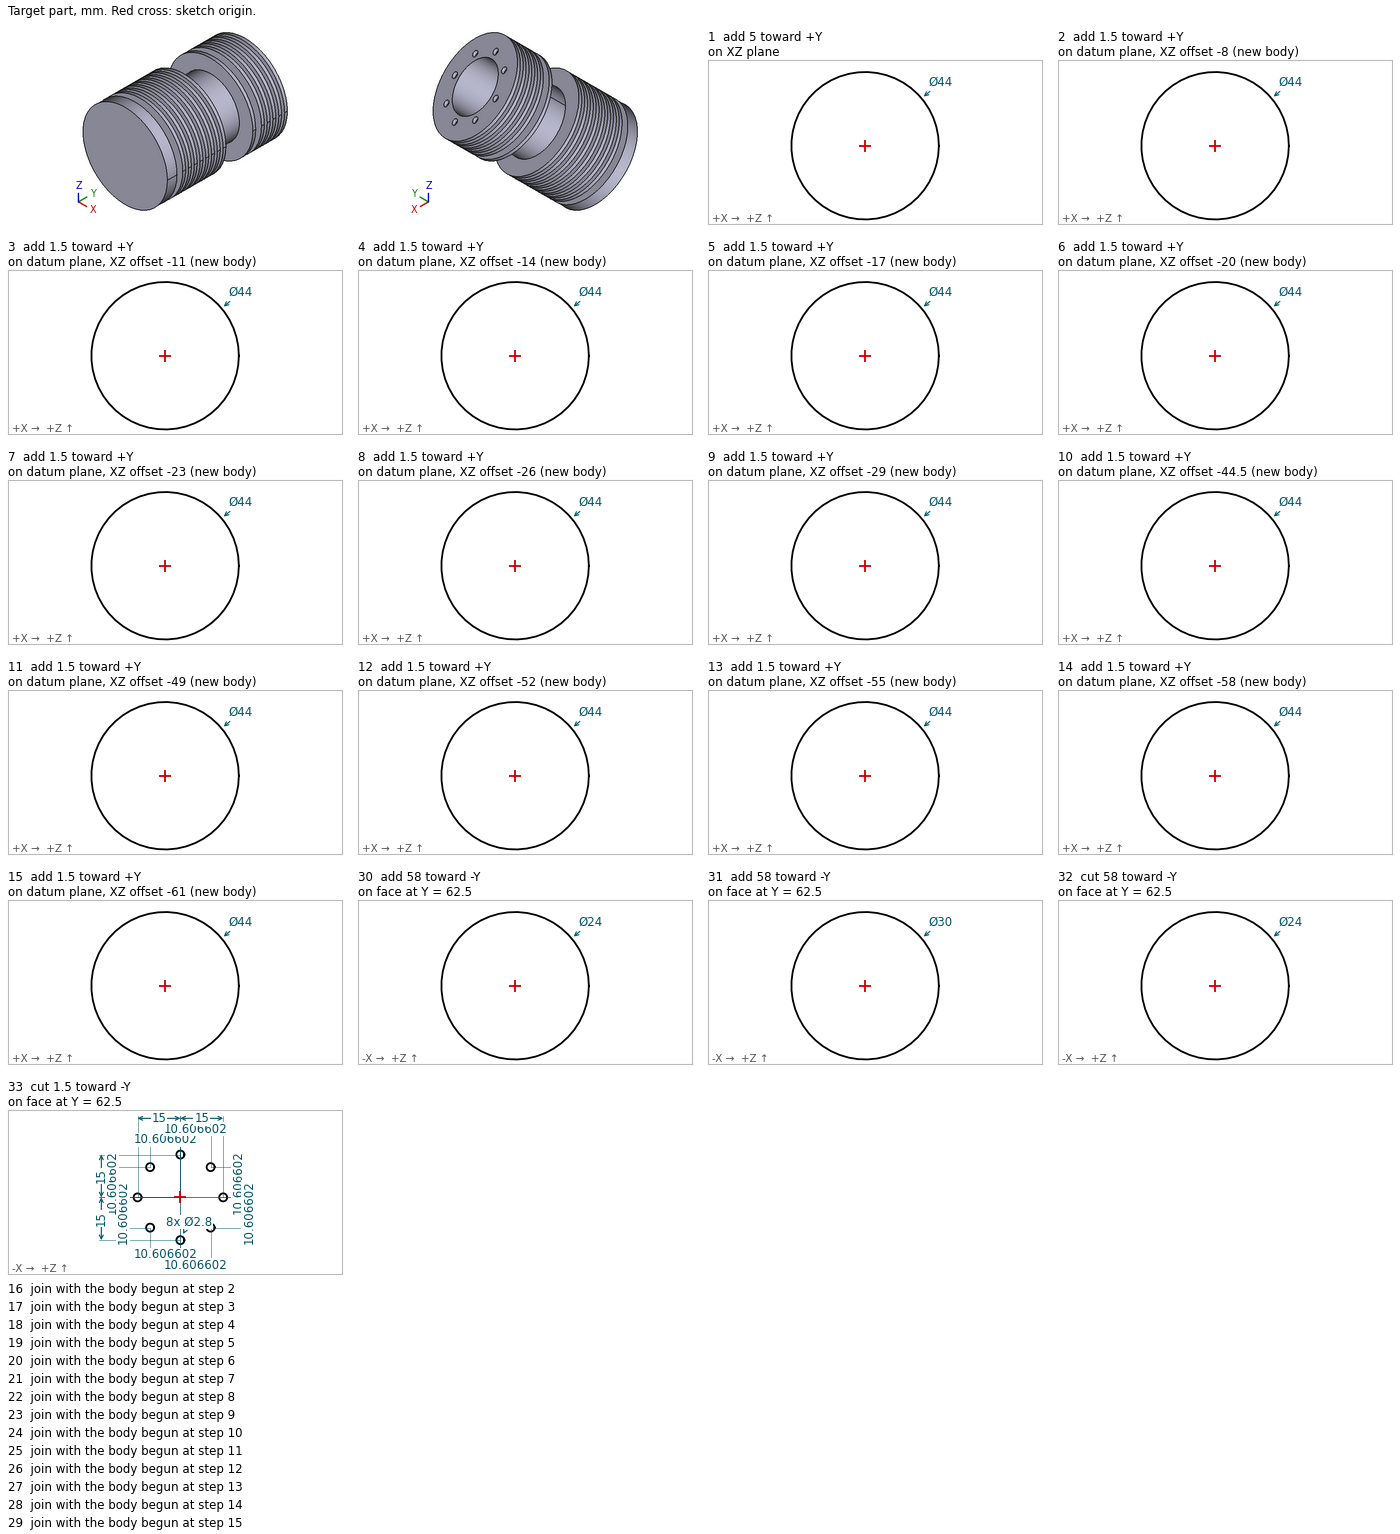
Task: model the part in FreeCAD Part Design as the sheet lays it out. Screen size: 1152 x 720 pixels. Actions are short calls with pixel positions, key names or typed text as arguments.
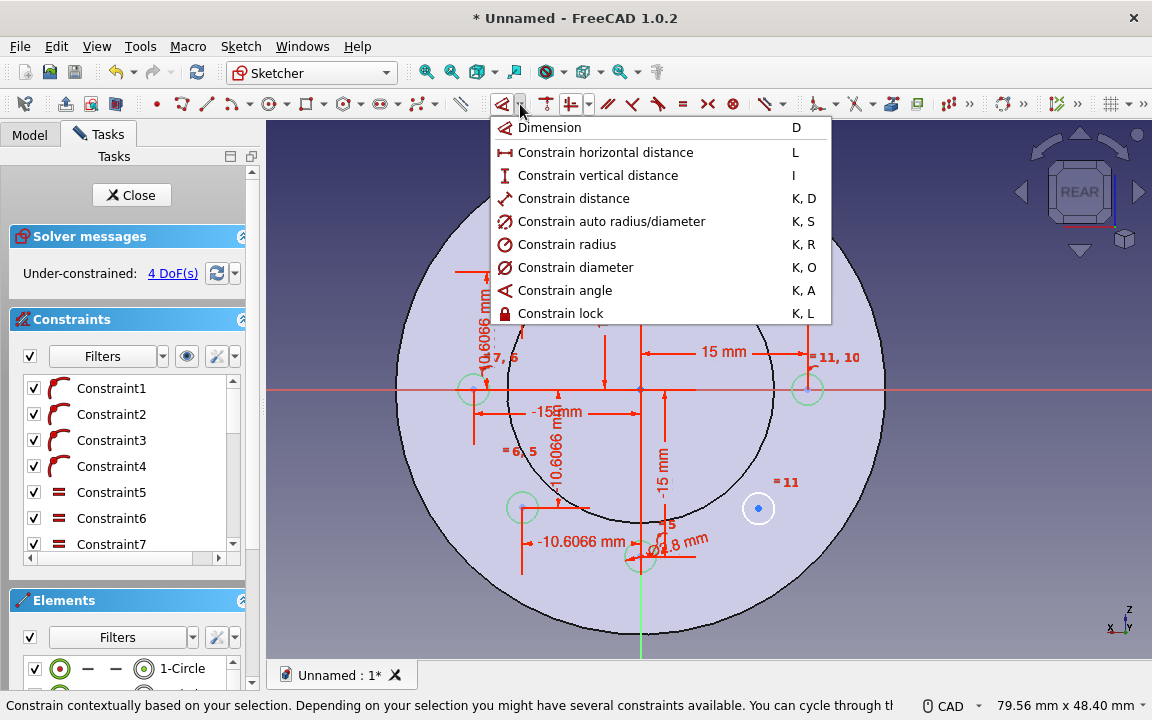
click(661, 152)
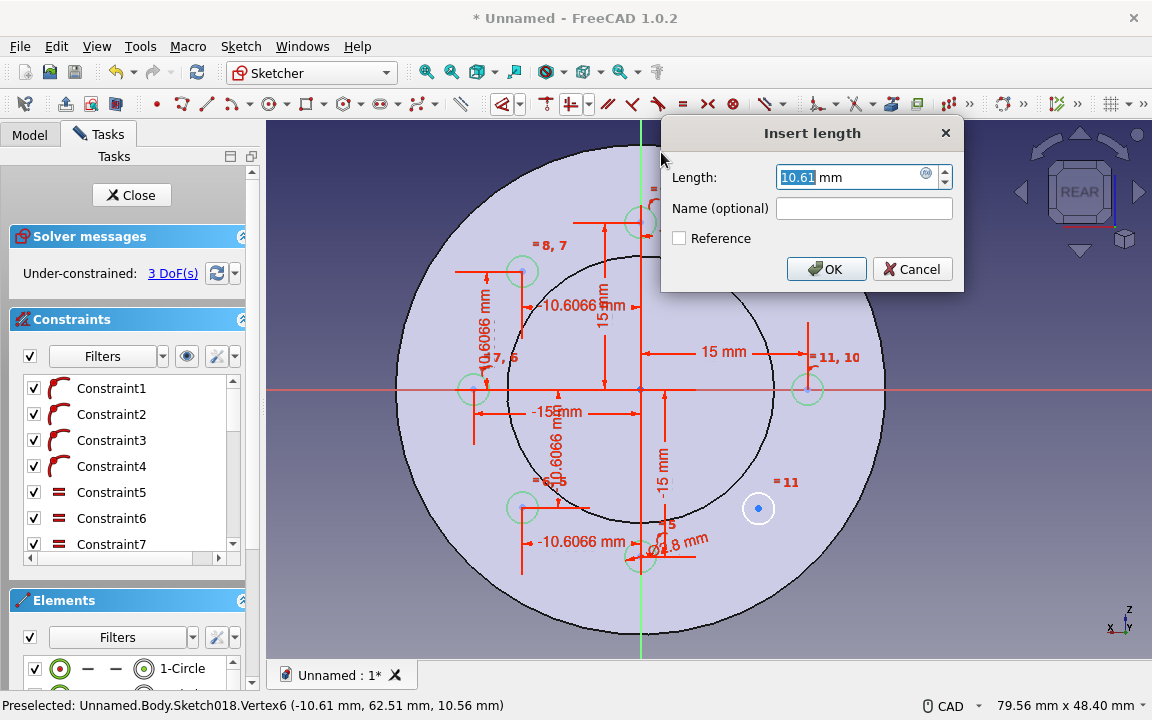
text(10.606602)
key(Return)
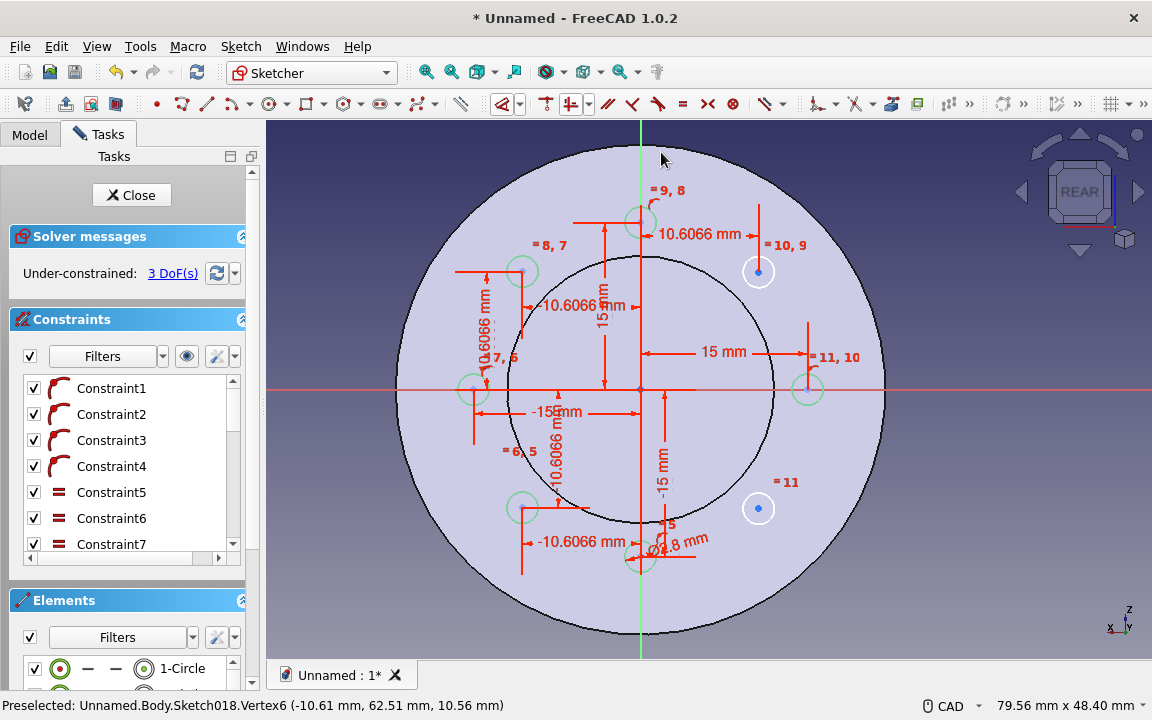
click(759, 272)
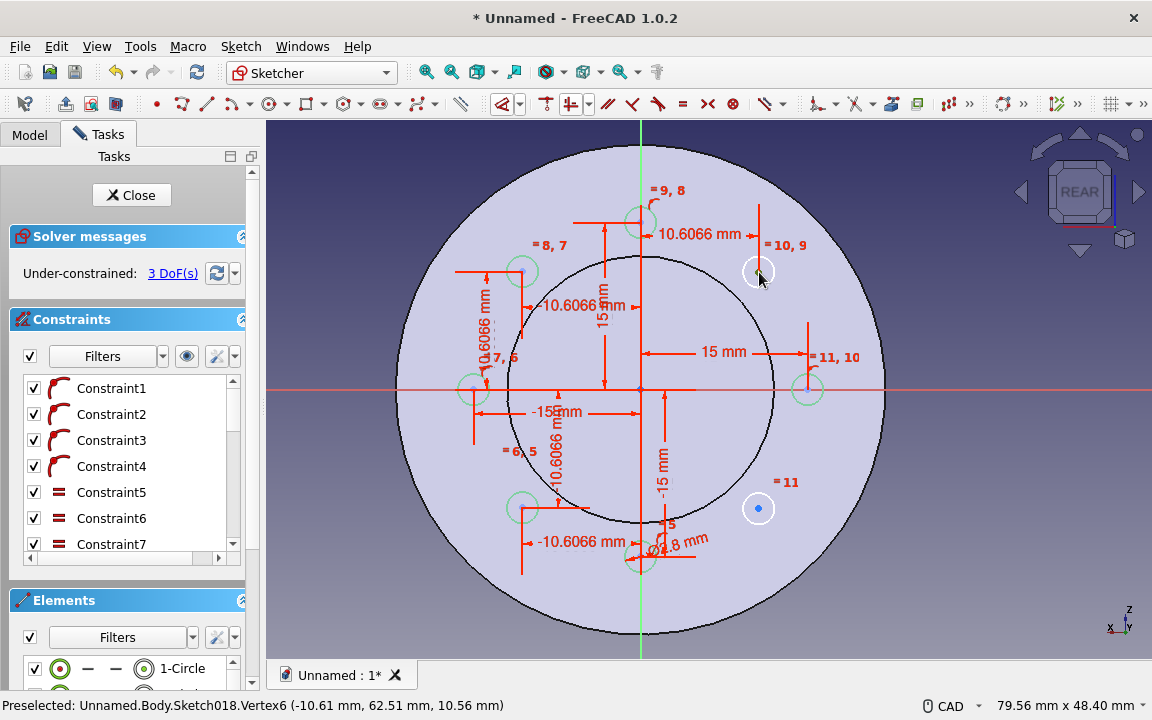
key(i)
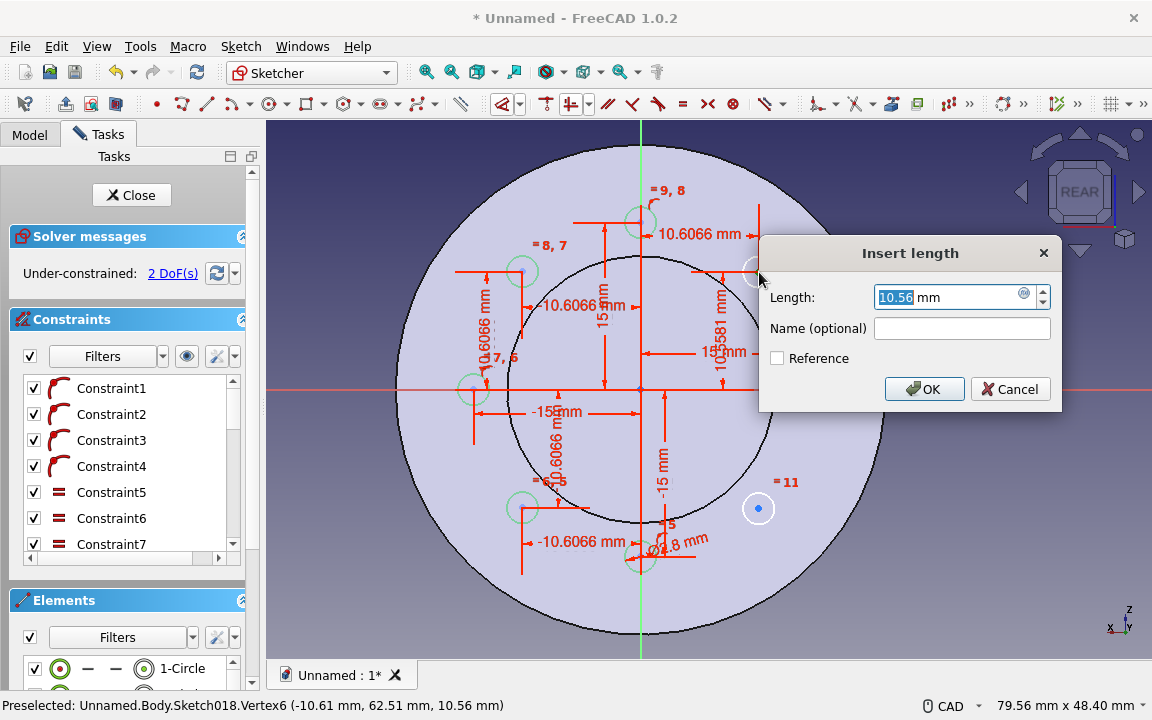
text(10.606602)
key(Return)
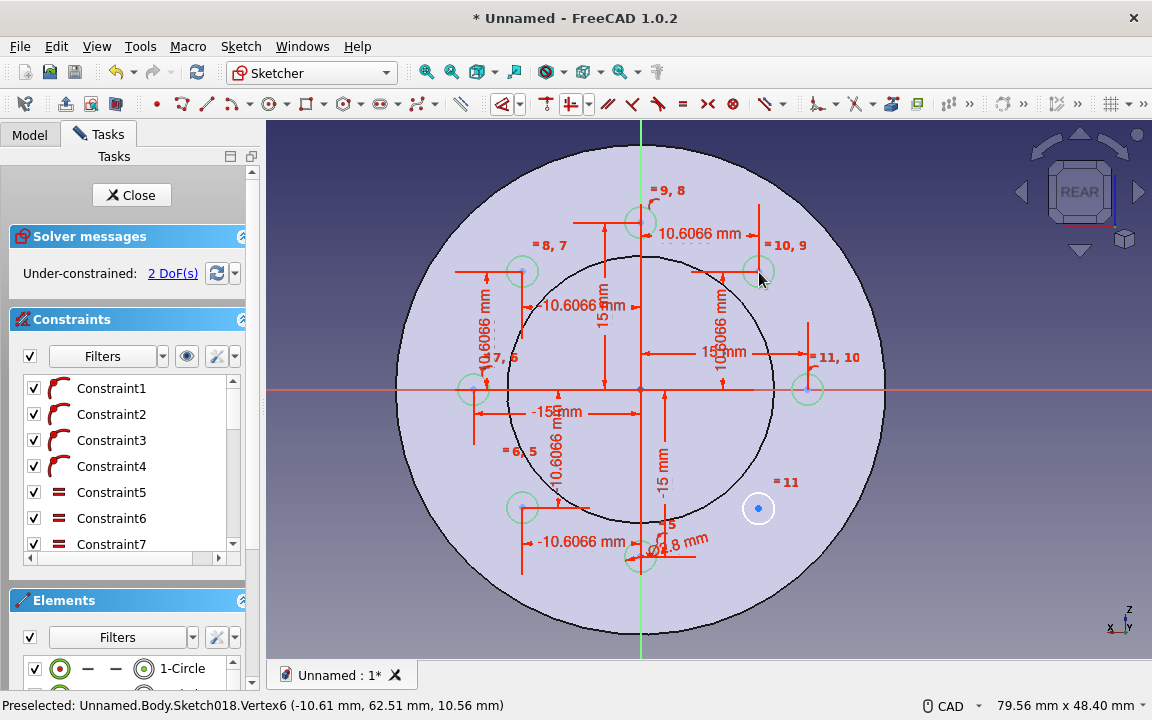
click(759, 509)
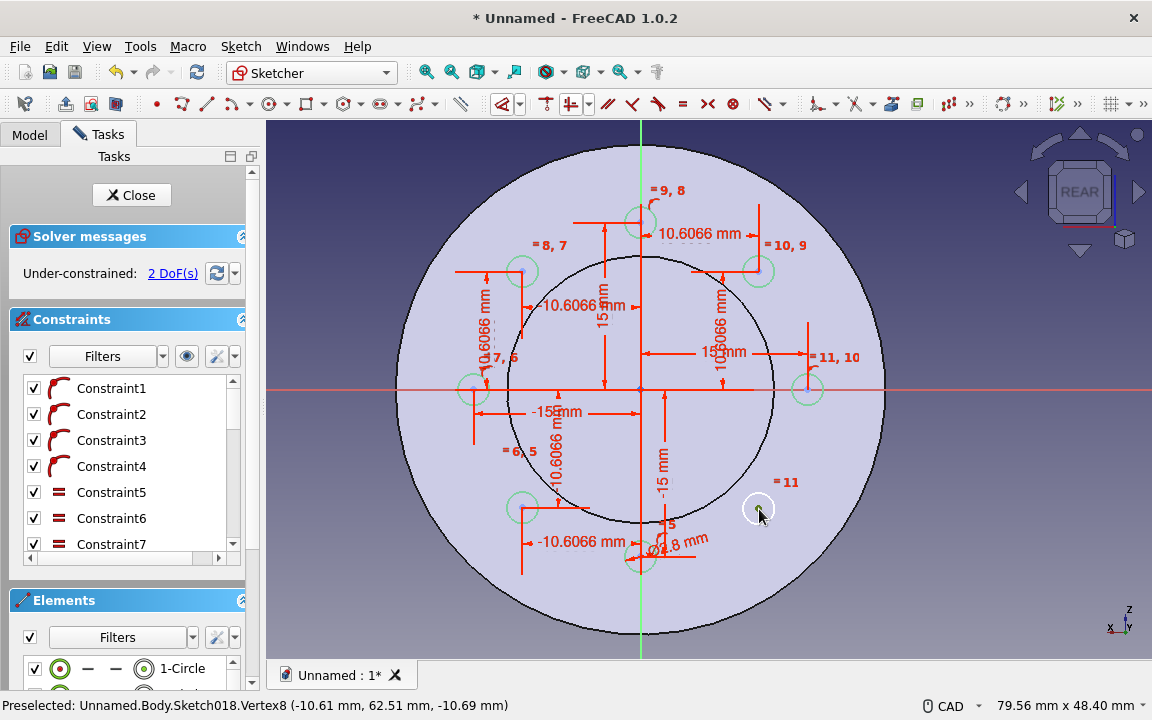
key(l)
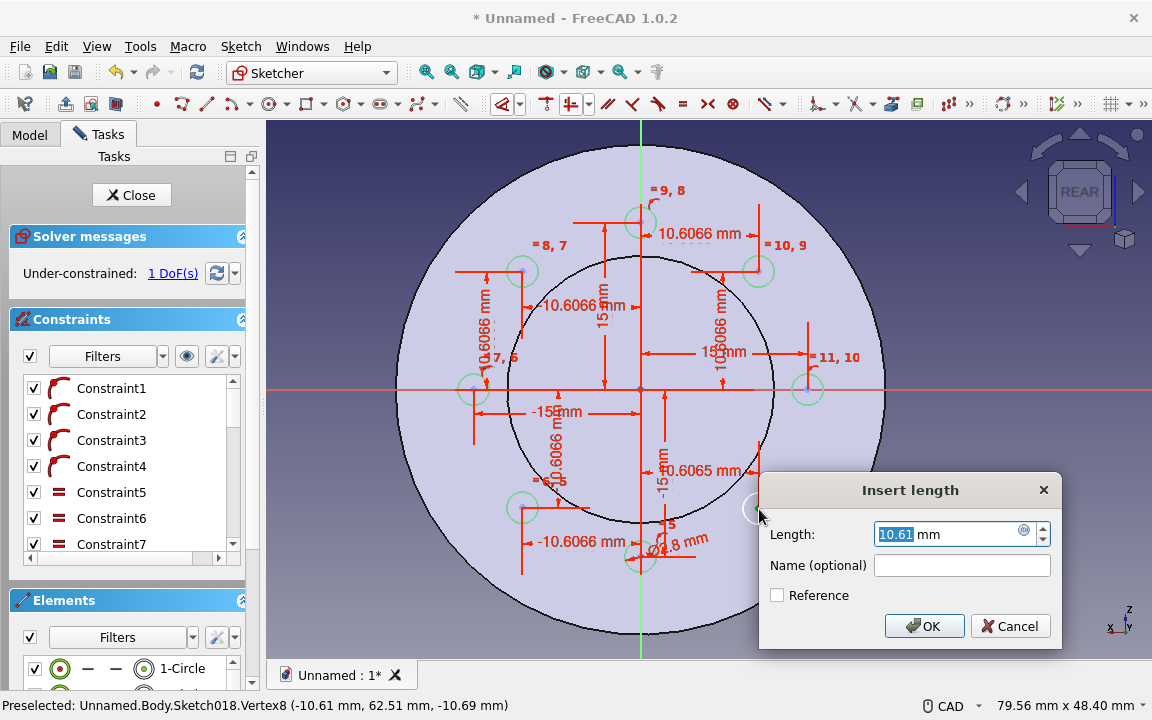
text(10.606602)
key(Return)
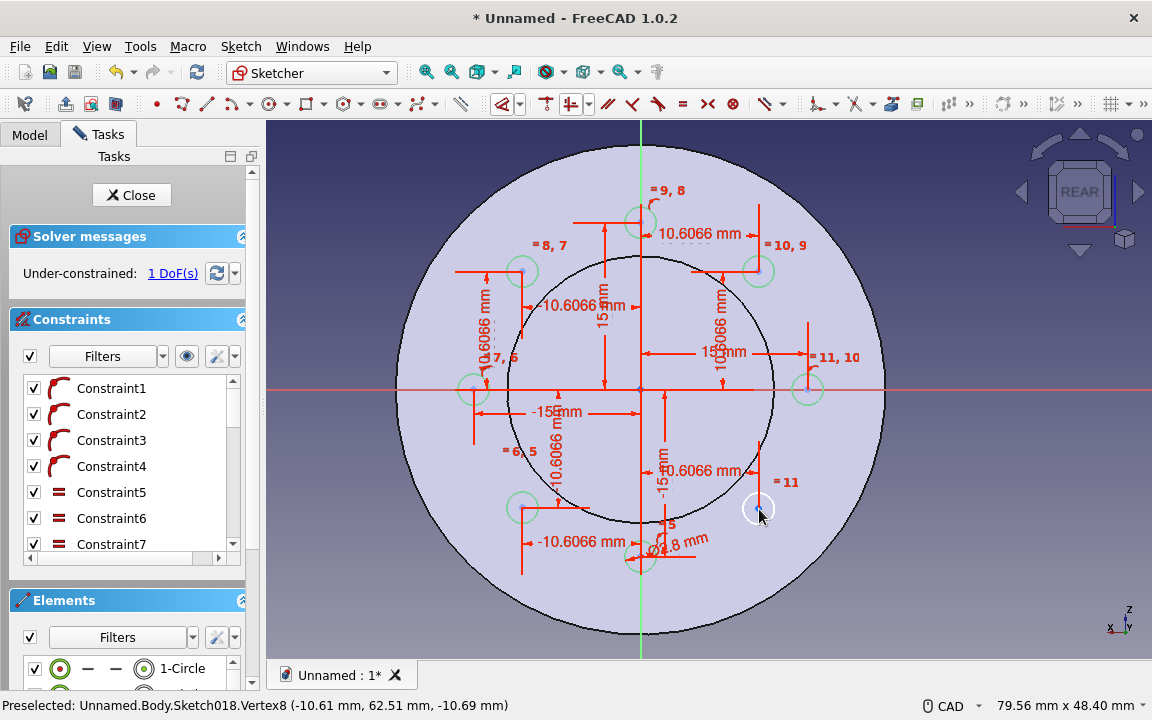
click(759, 509)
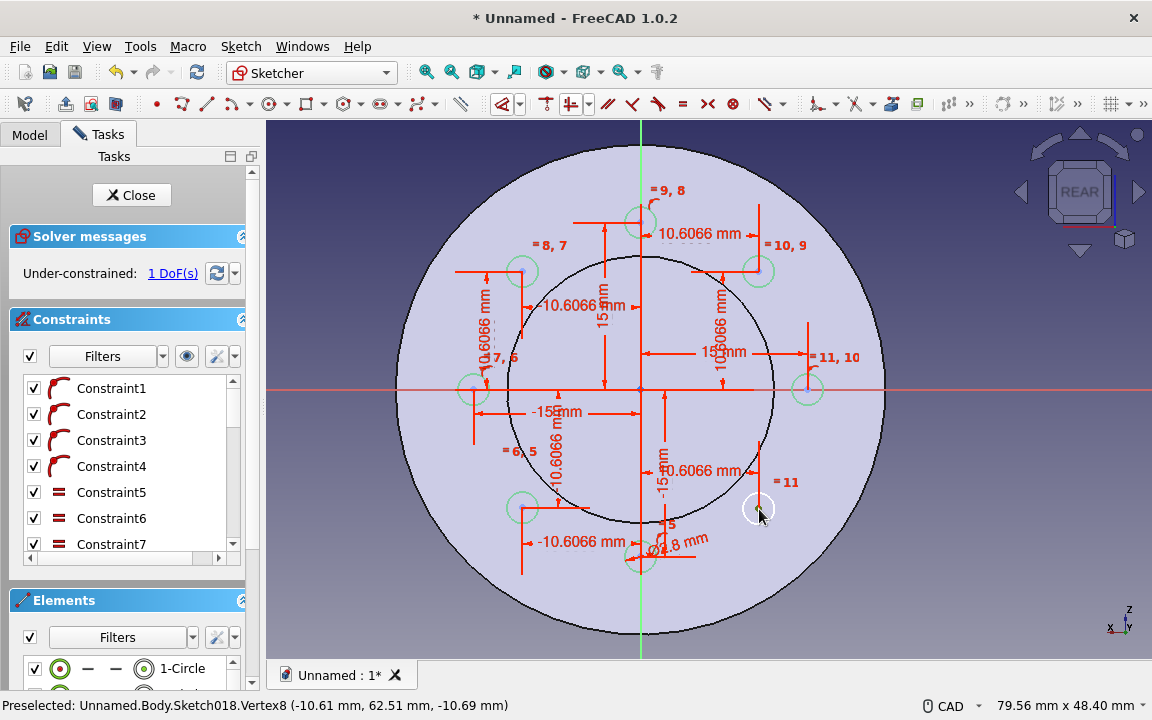
key(i)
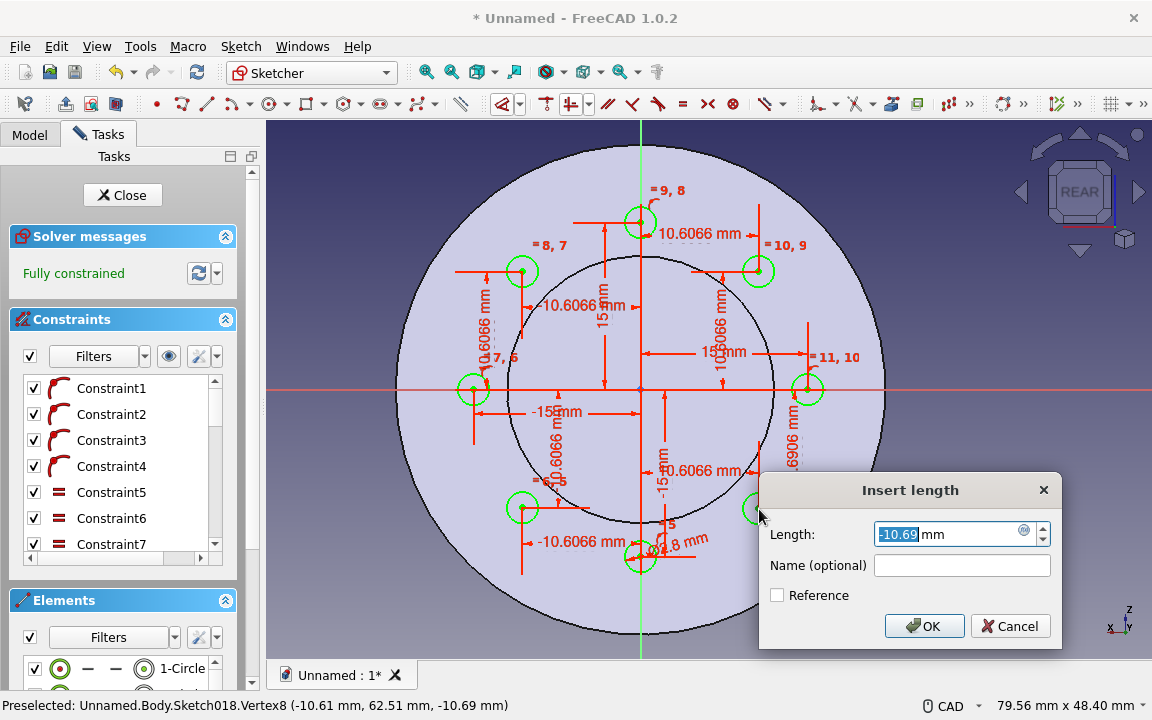
text(-10.606602)
key(Return)